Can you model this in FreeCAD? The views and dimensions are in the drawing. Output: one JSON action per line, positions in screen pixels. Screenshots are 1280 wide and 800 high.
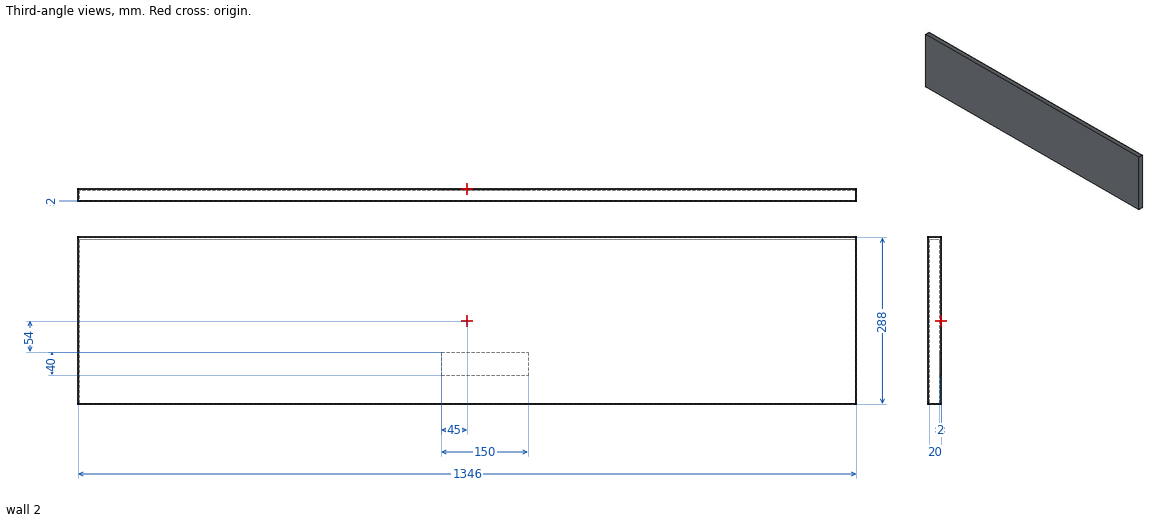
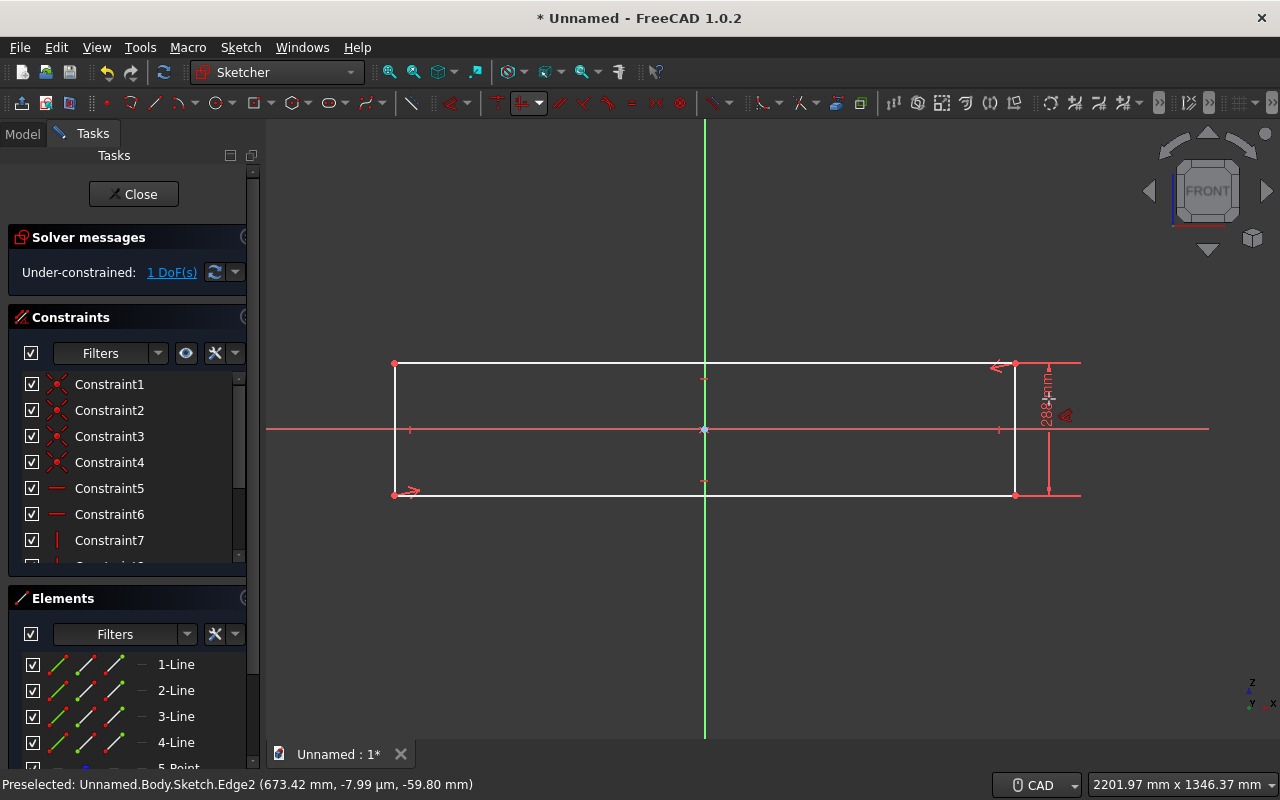
{"action": "left_click", "coordinate": [581, 496]}
{"action": "left_click", "coordinate": [562, 530]}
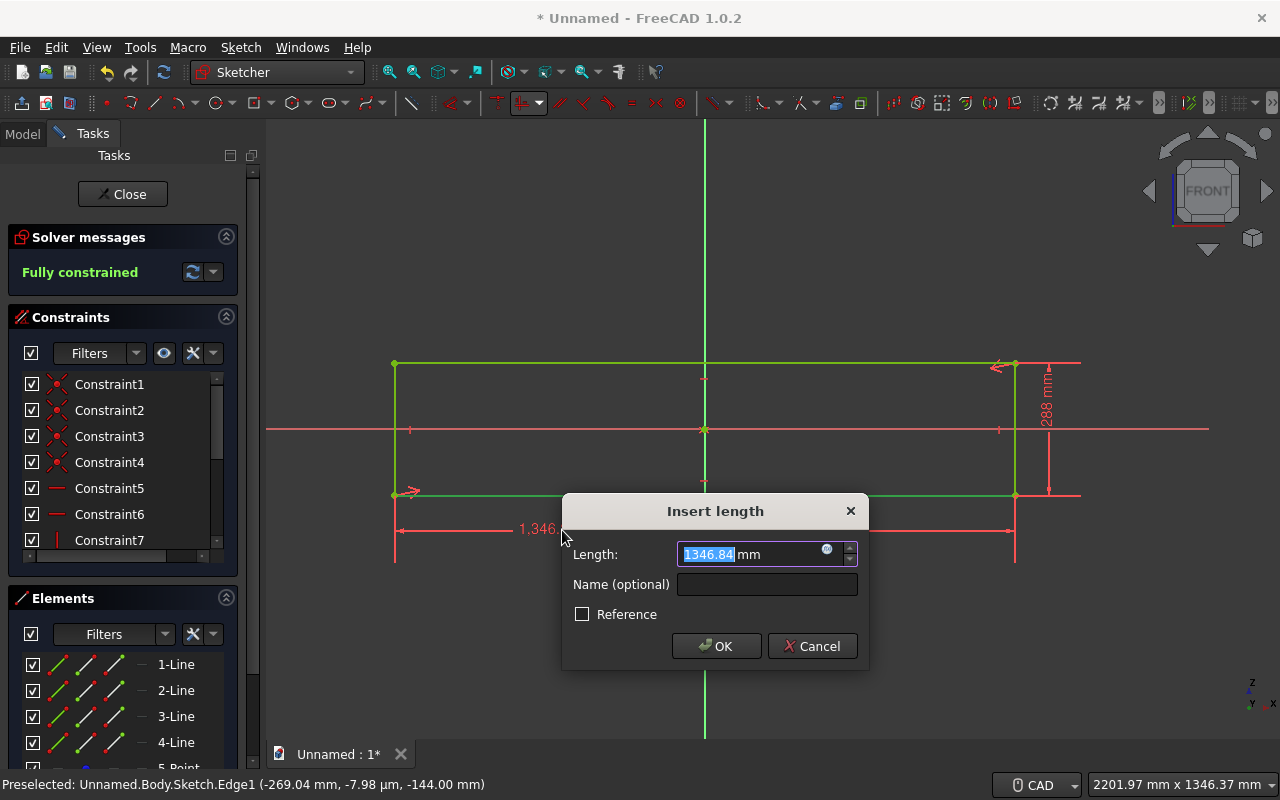
{"action": "type", "text": "1346"}
{"action": "key", "text": "Return"}
{"action": "key", "text": "Escape"}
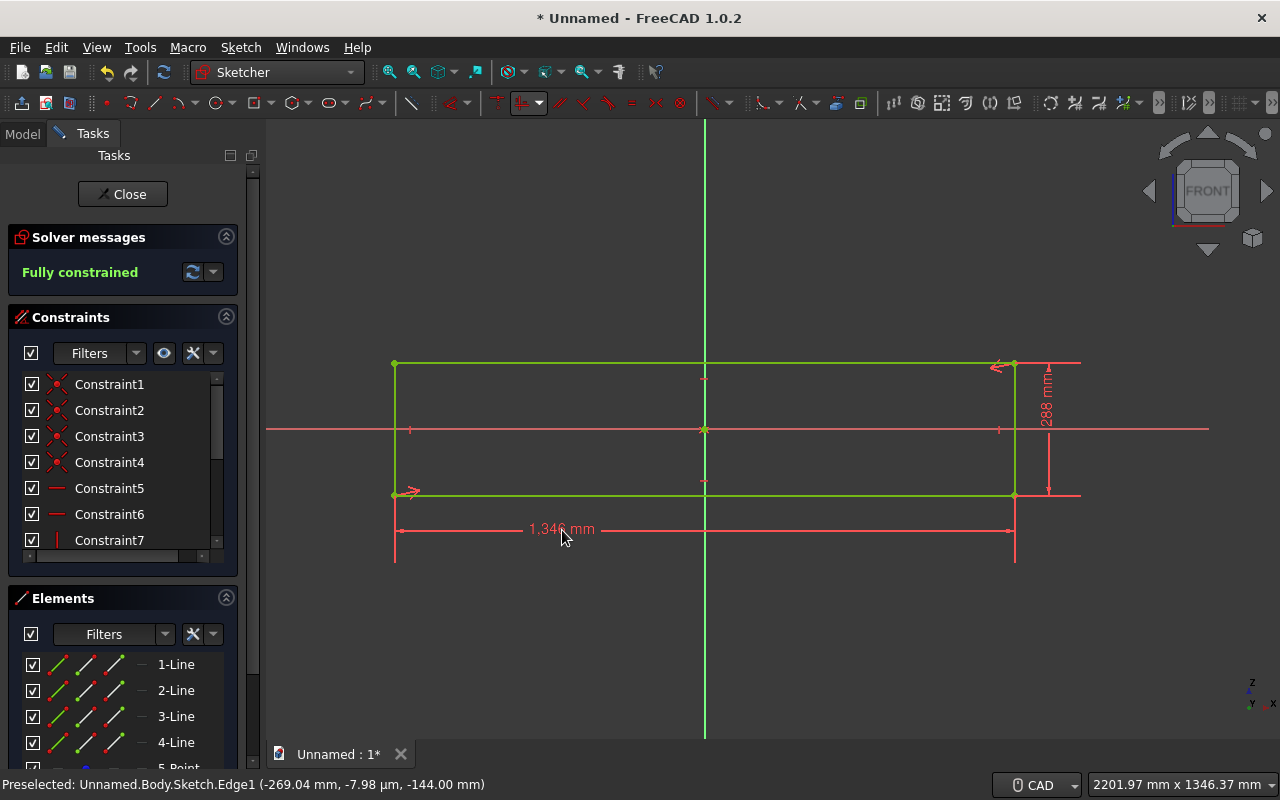
{"action": "left_click", "coordinate": [123, 194]}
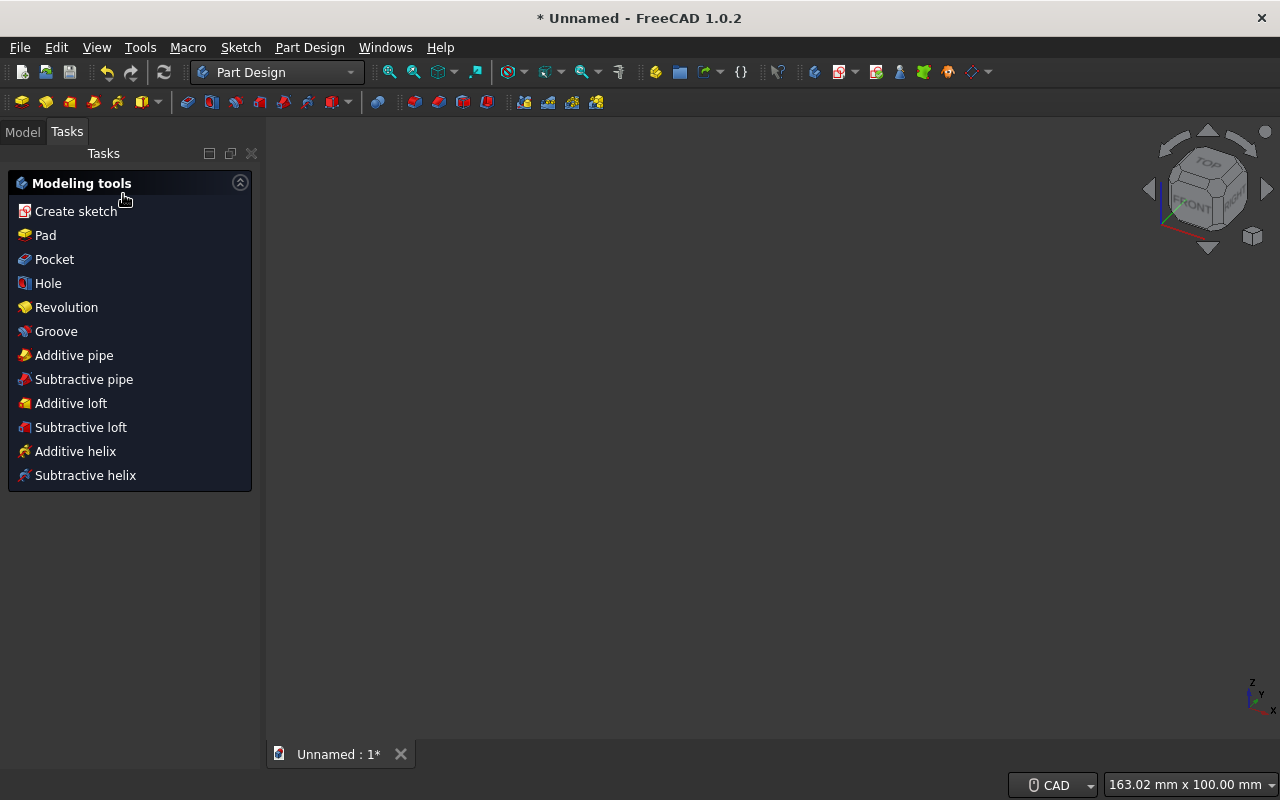
{"action": "left_click", "coordinate": [22, 102]}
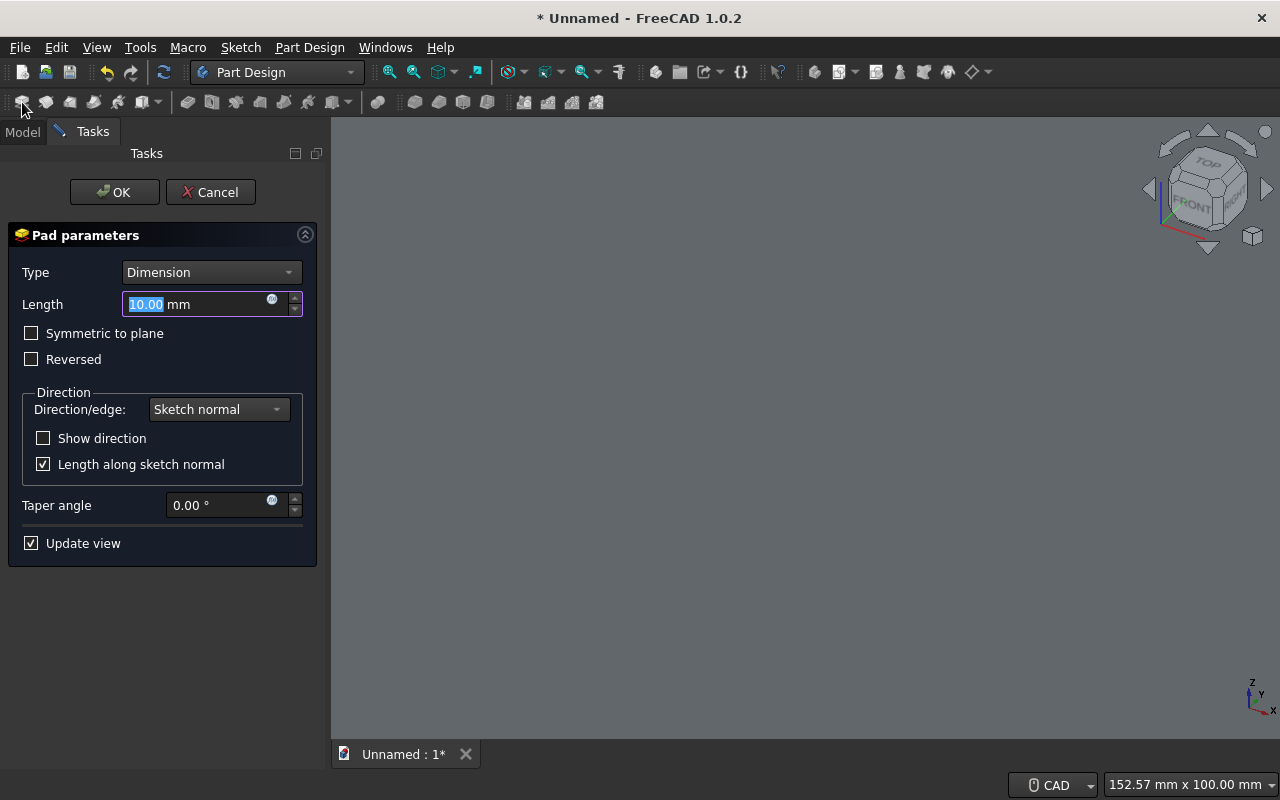
{"action": "type", "text": "20"}
{"action": "key", "text": "Tab"}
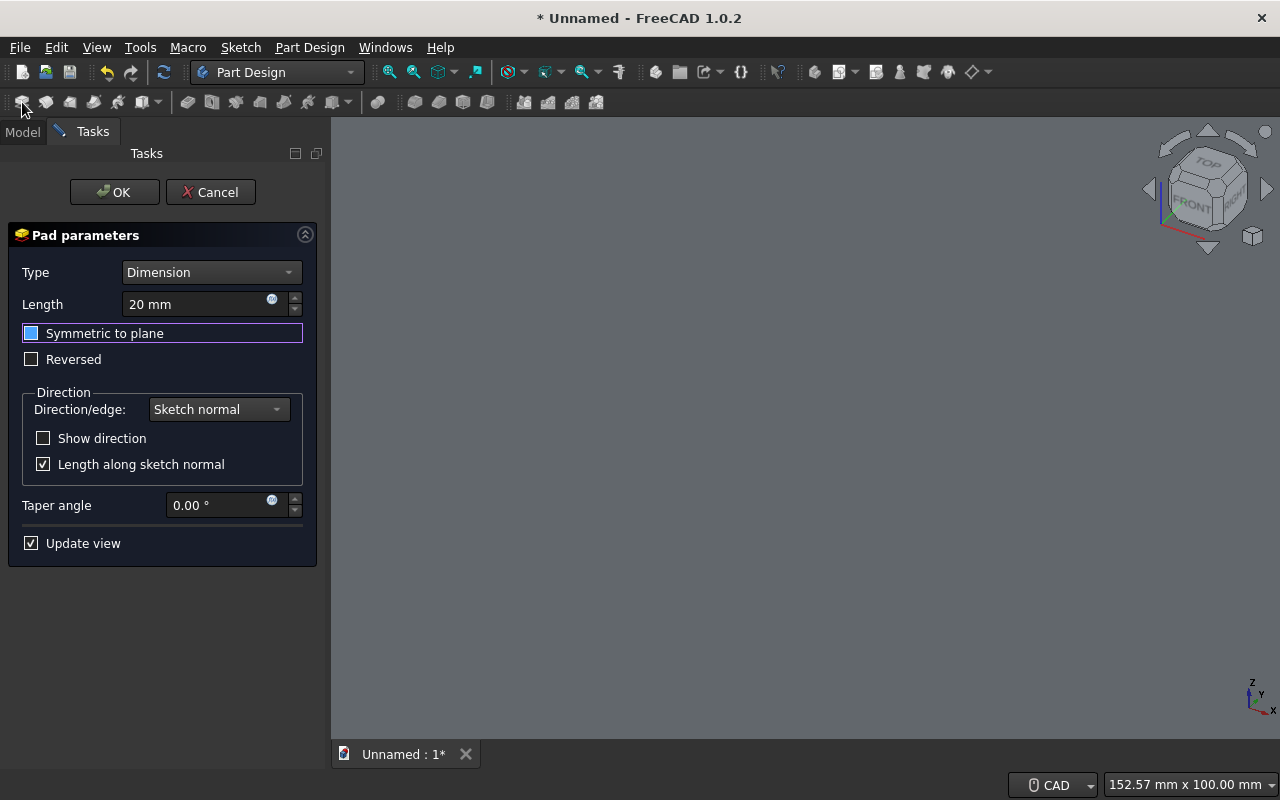
{"action": "left_click", "coordinate": [115, 192]}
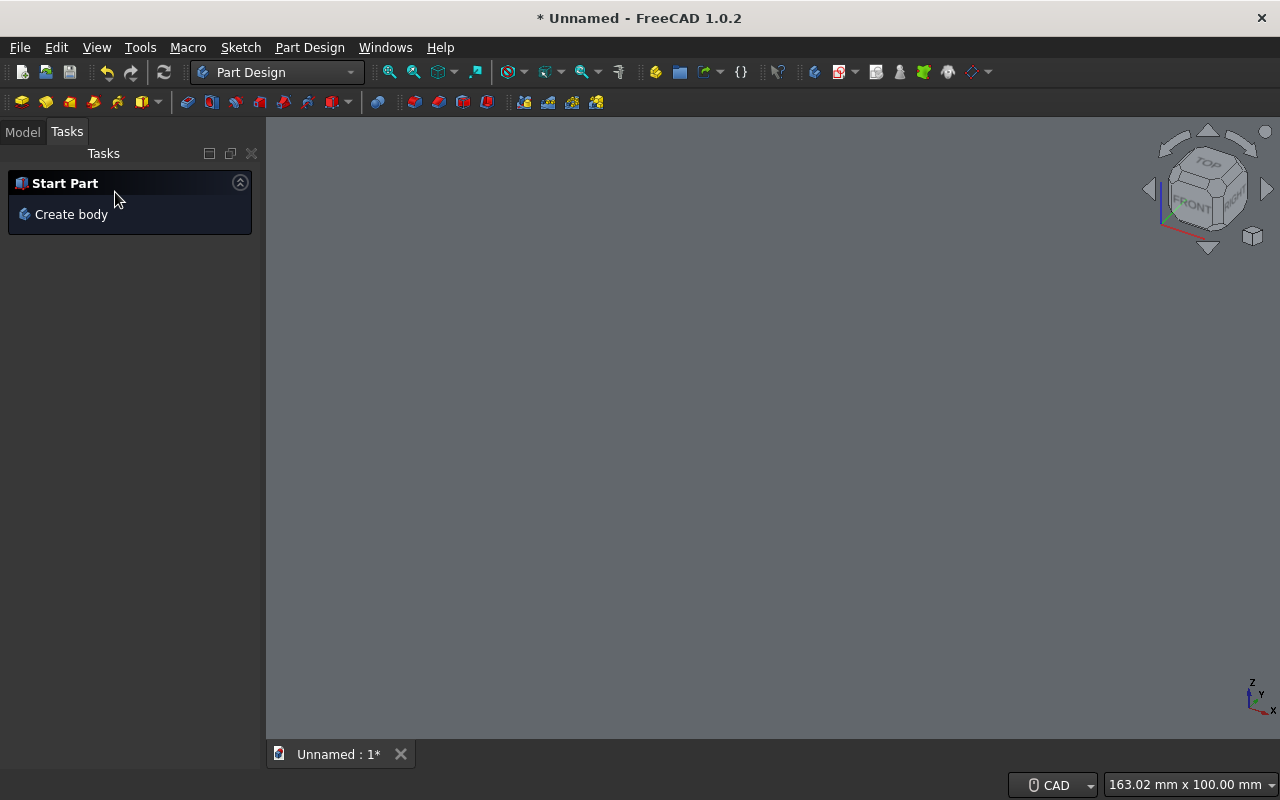
{"action": "key", "text": "v f"}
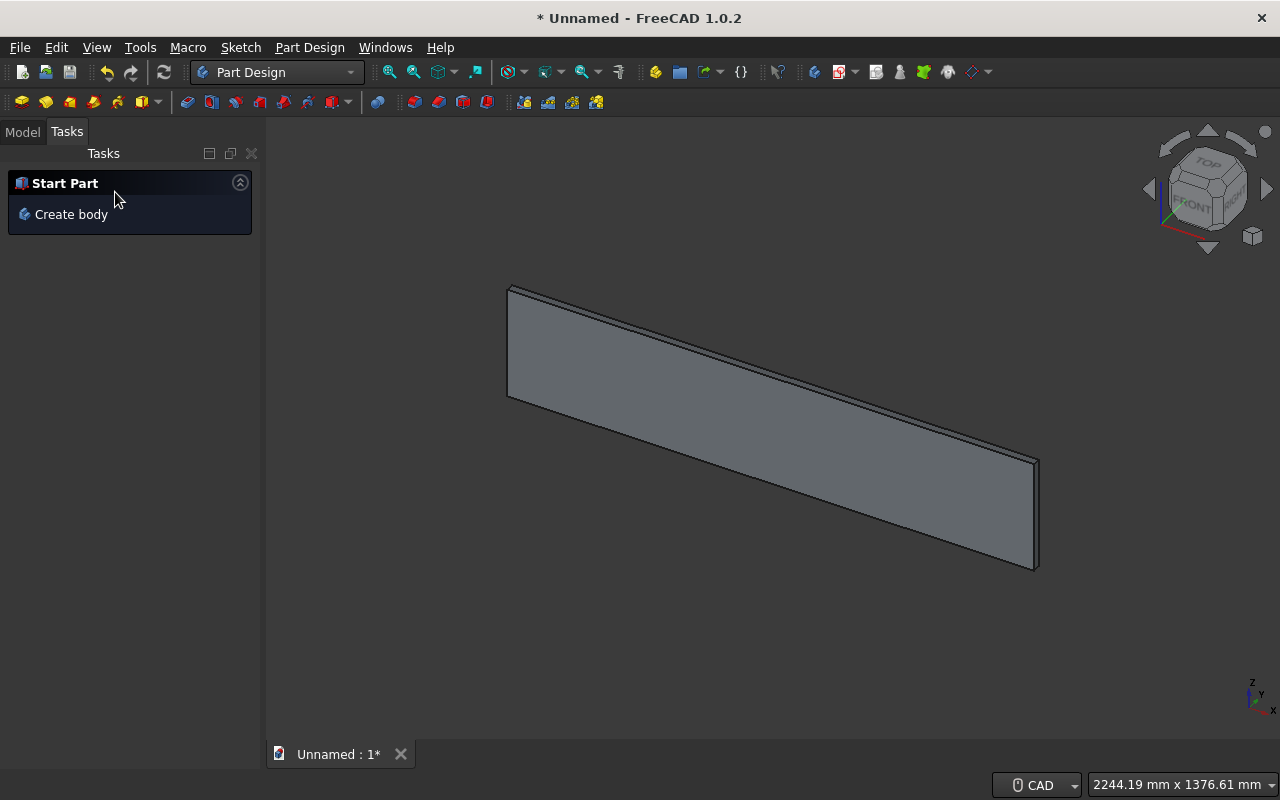
{"action": "left_click", "coordinate": [921, 479]}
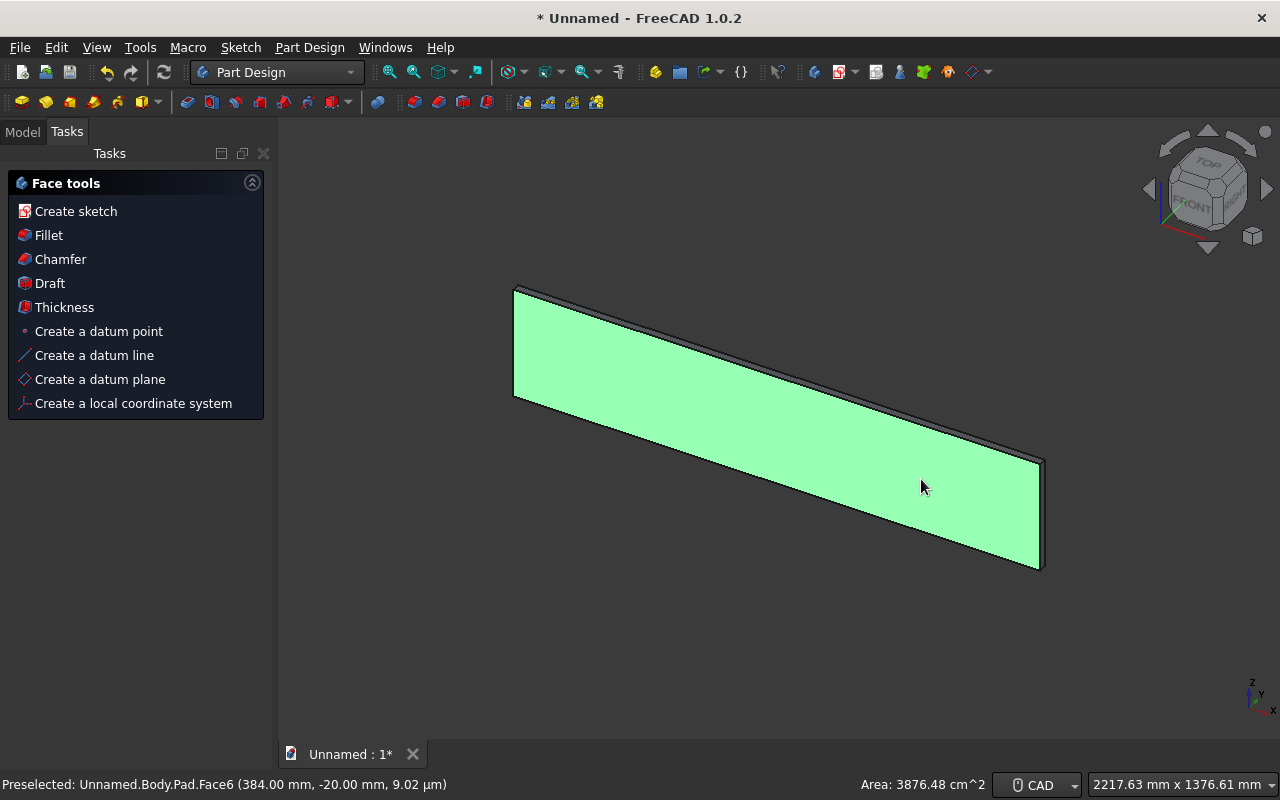
{"action": "left_click", "coordinate": [488, 102]}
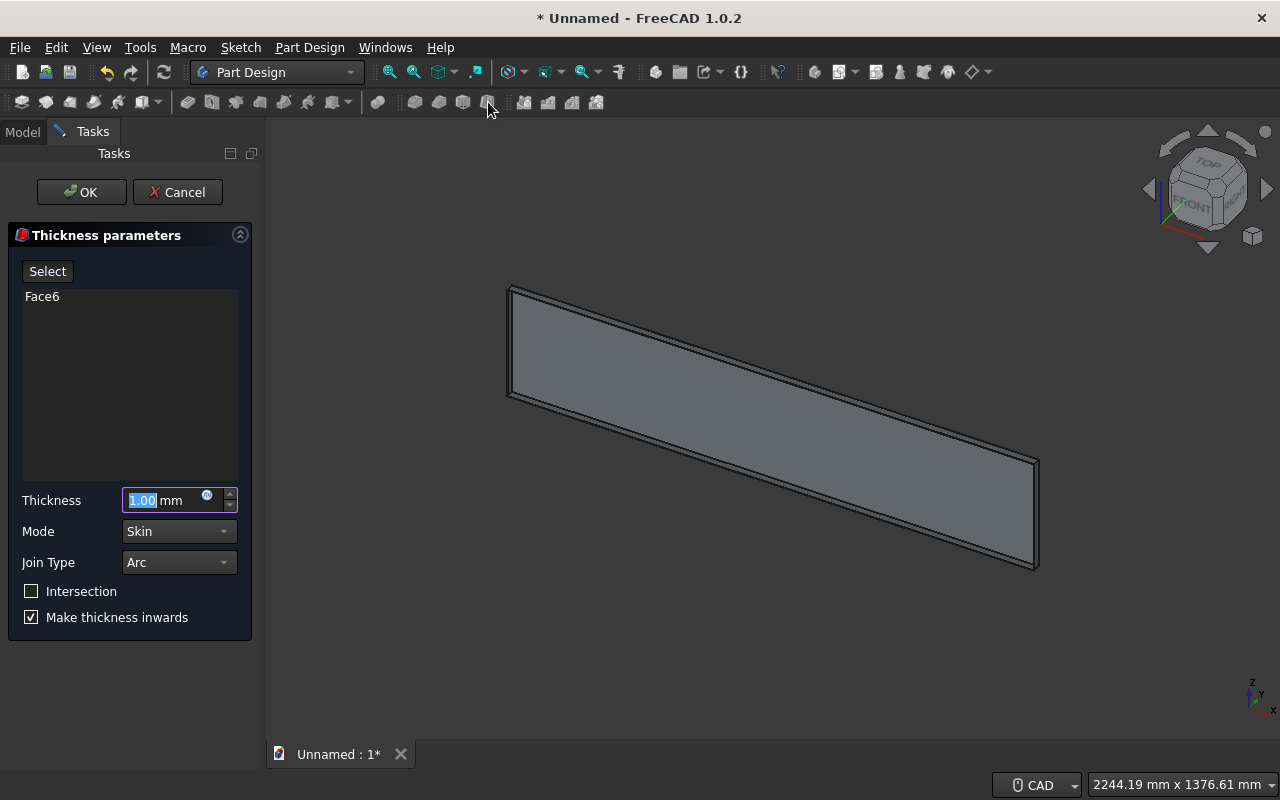
{"action": "type", "text": "2"}
{"action": "key", "text": "Tab"}